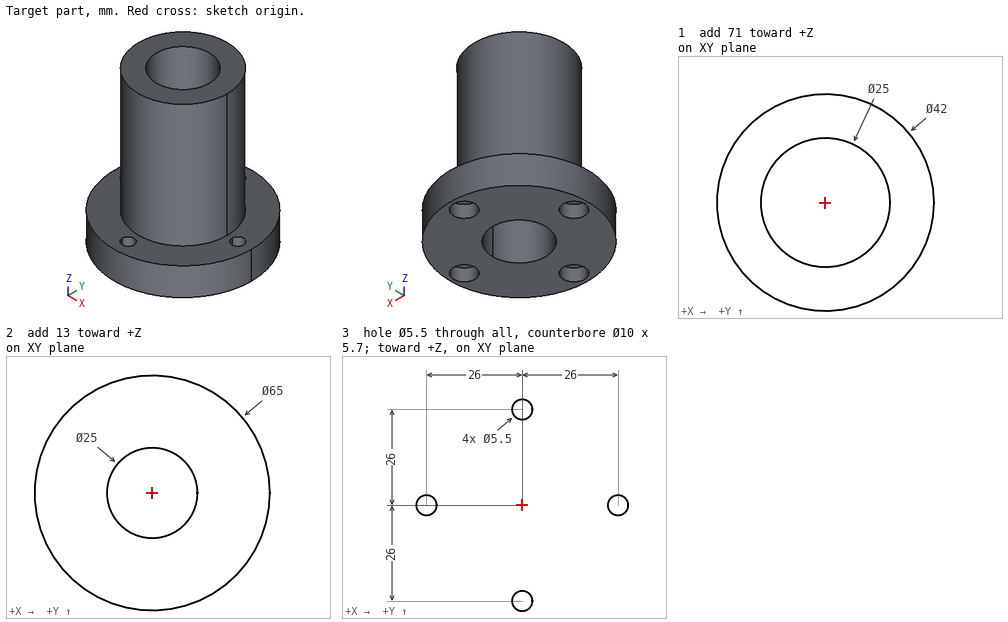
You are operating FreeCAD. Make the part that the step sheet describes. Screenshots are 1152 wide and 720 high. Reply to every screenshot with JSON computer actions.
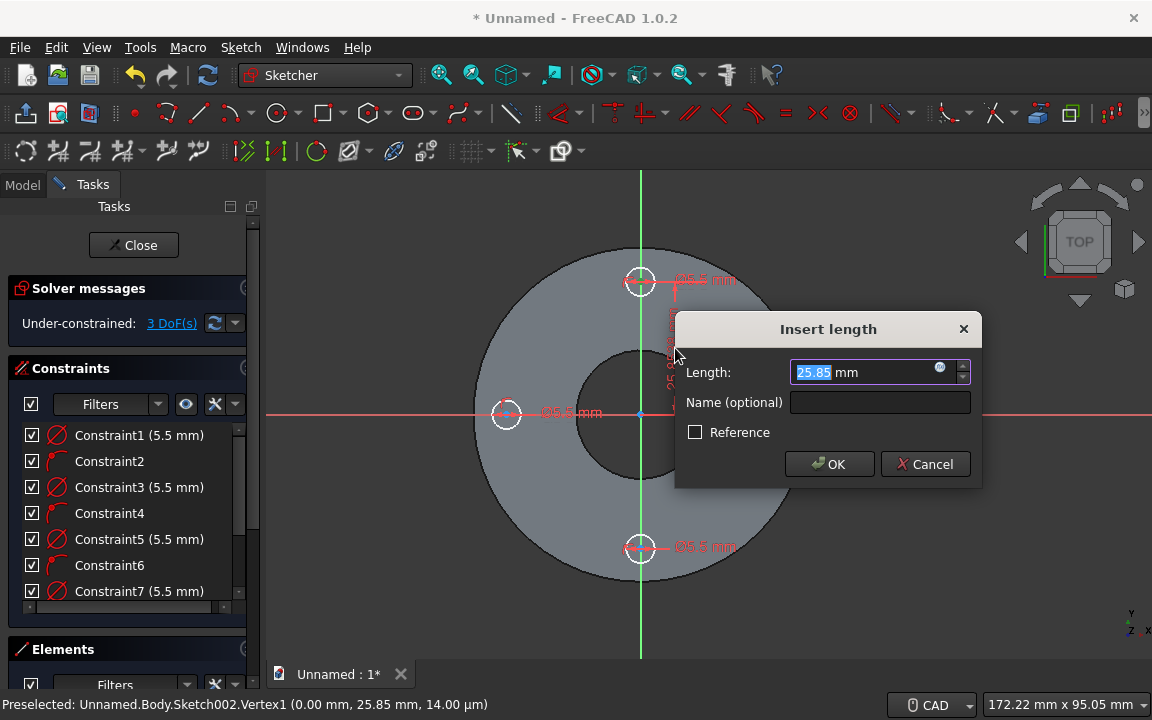
{"action": "type", "text": "26"}
{"action": "key", "text": "Return"}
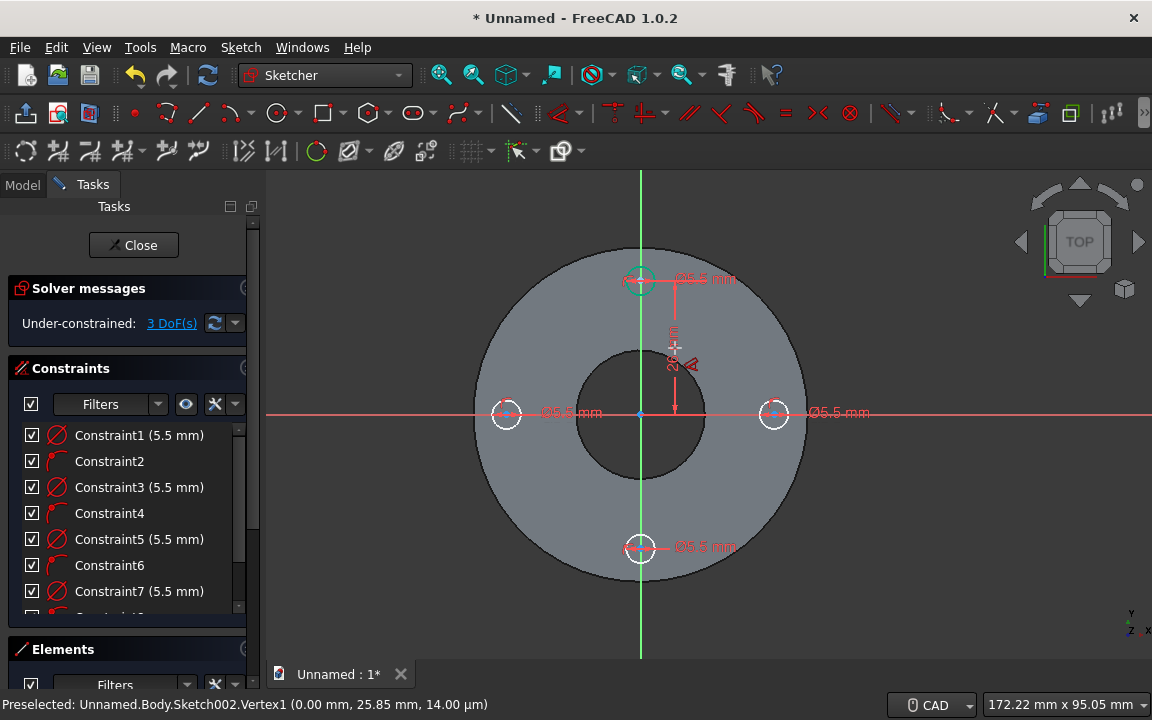
{"action": "left_click", "coordinate": [507, 415]}
{"action": "left_click", "coordinate": [574, 449]}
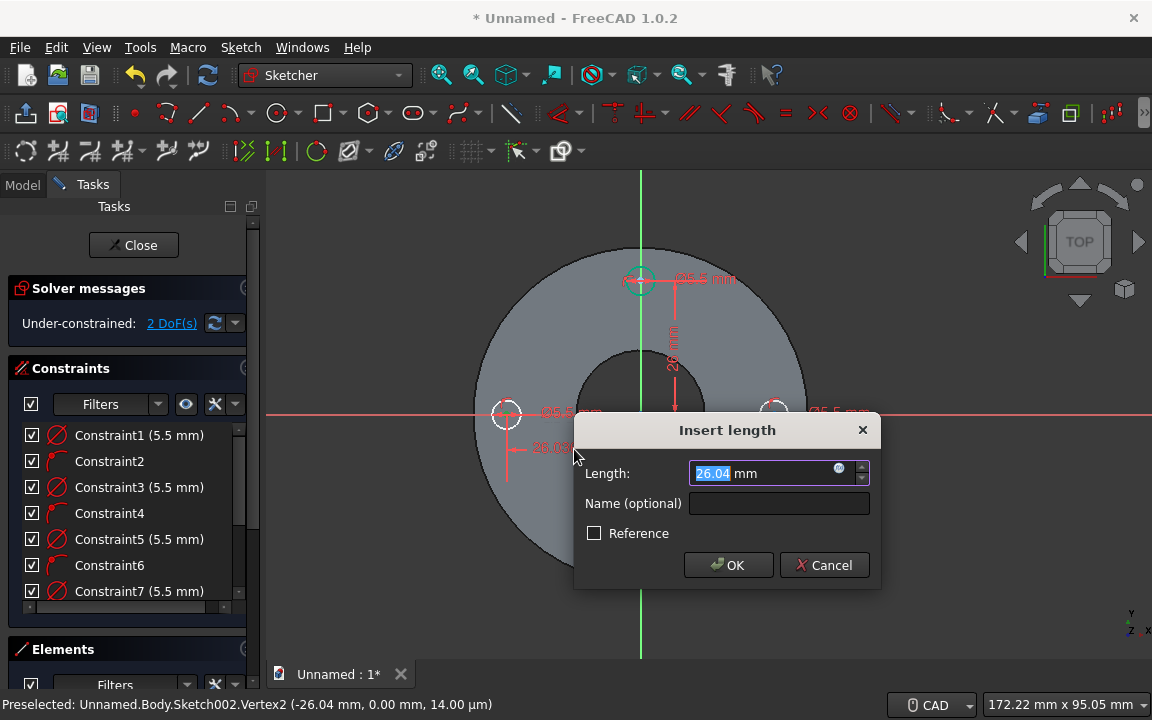
{"action": "type", "text": "26"}
{"action": "key", "text": "Return"}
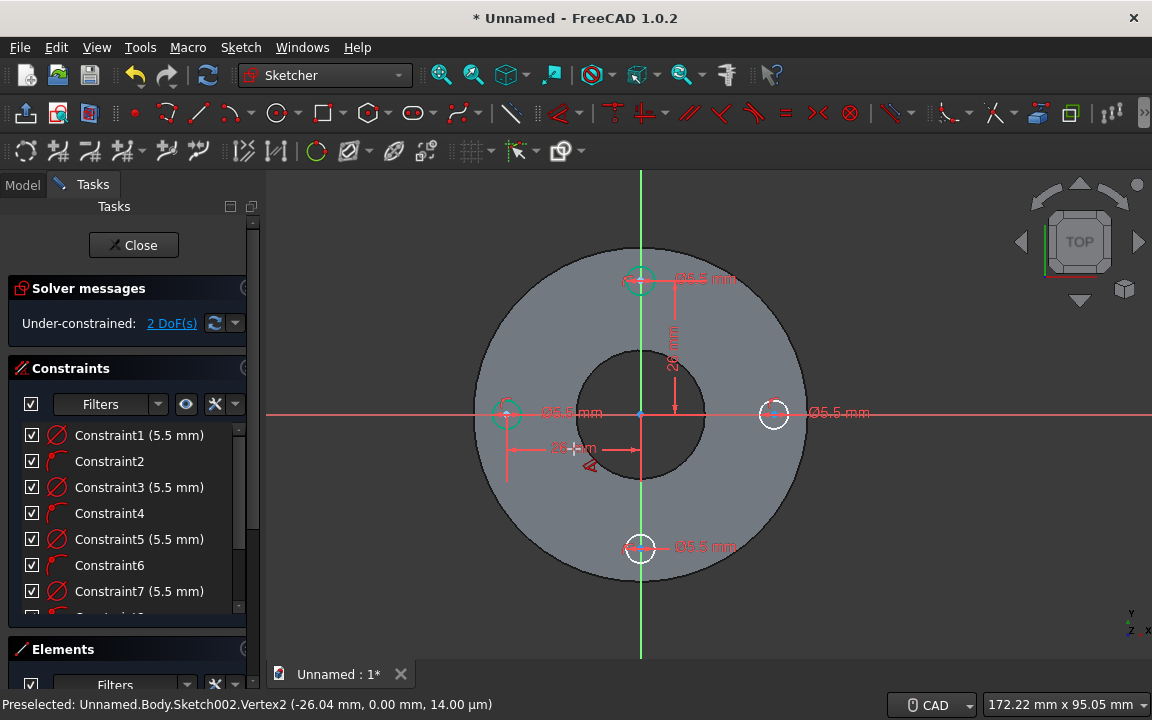
{"action": "left_click", "coordinate": [641, 549]}
{"action": "left_click", "coordinate": [675, 482]}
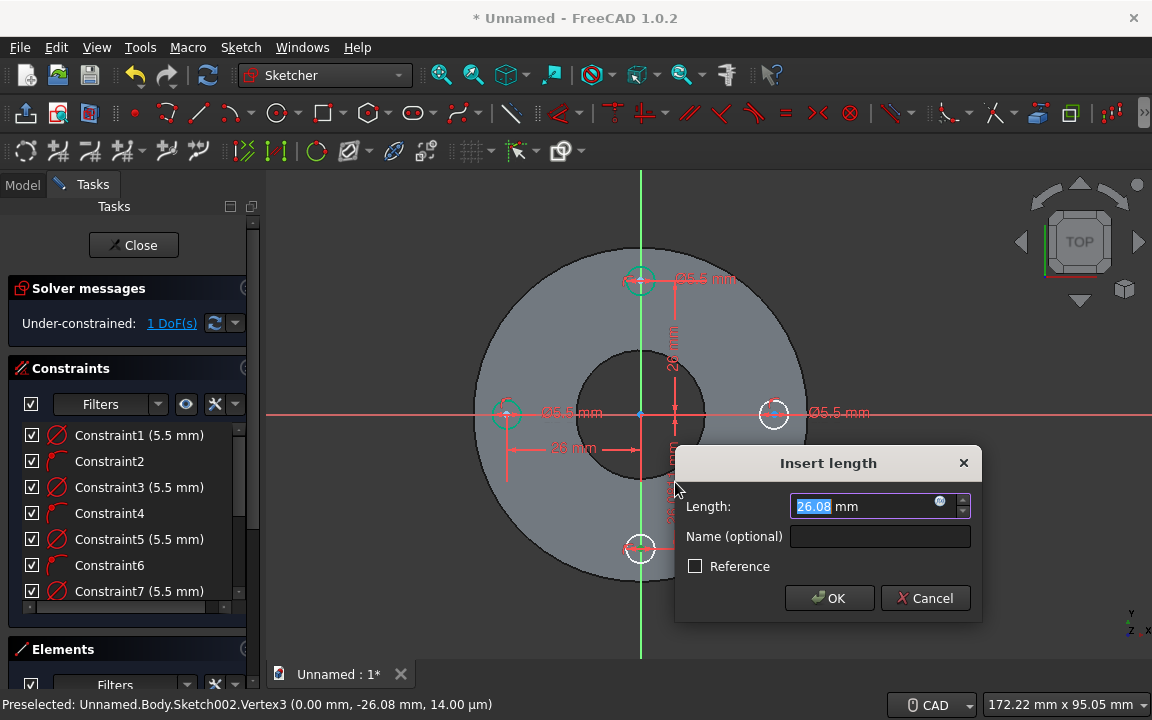
{"action": "type", "text": "26"}
{"action": "key", "text": "Return"}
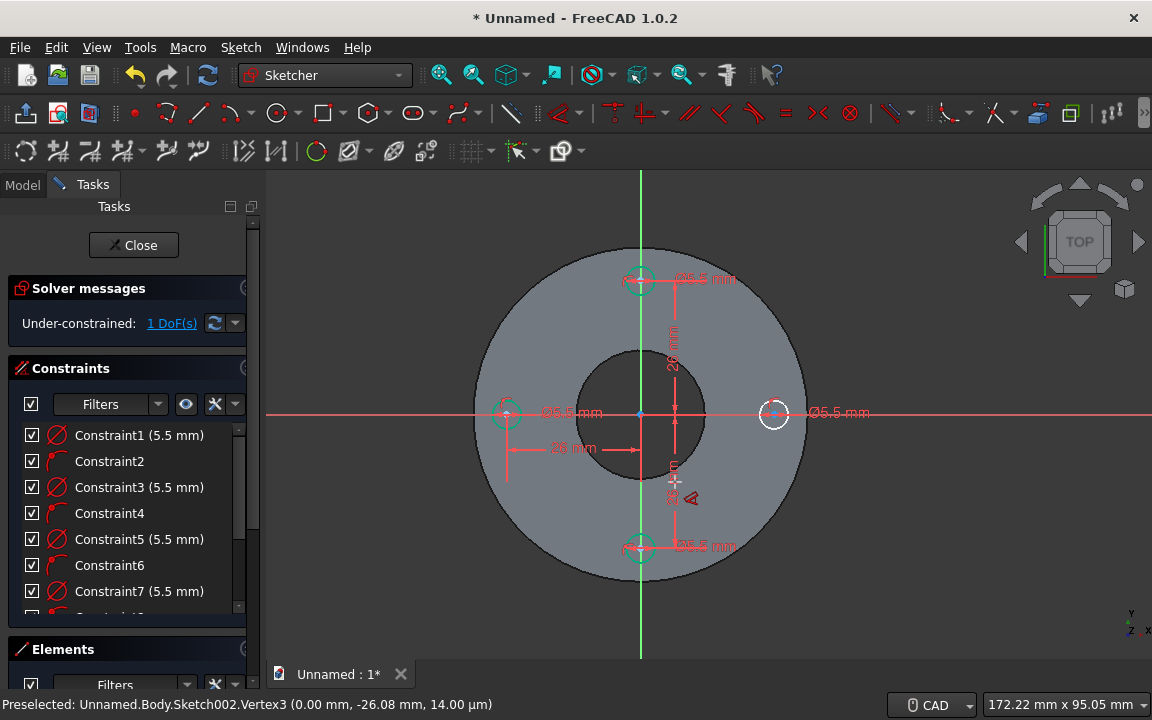
{"action": "left_click", "coordinate": [774, 415]}
{"action": "left_click", "coordinate": [707, 449]}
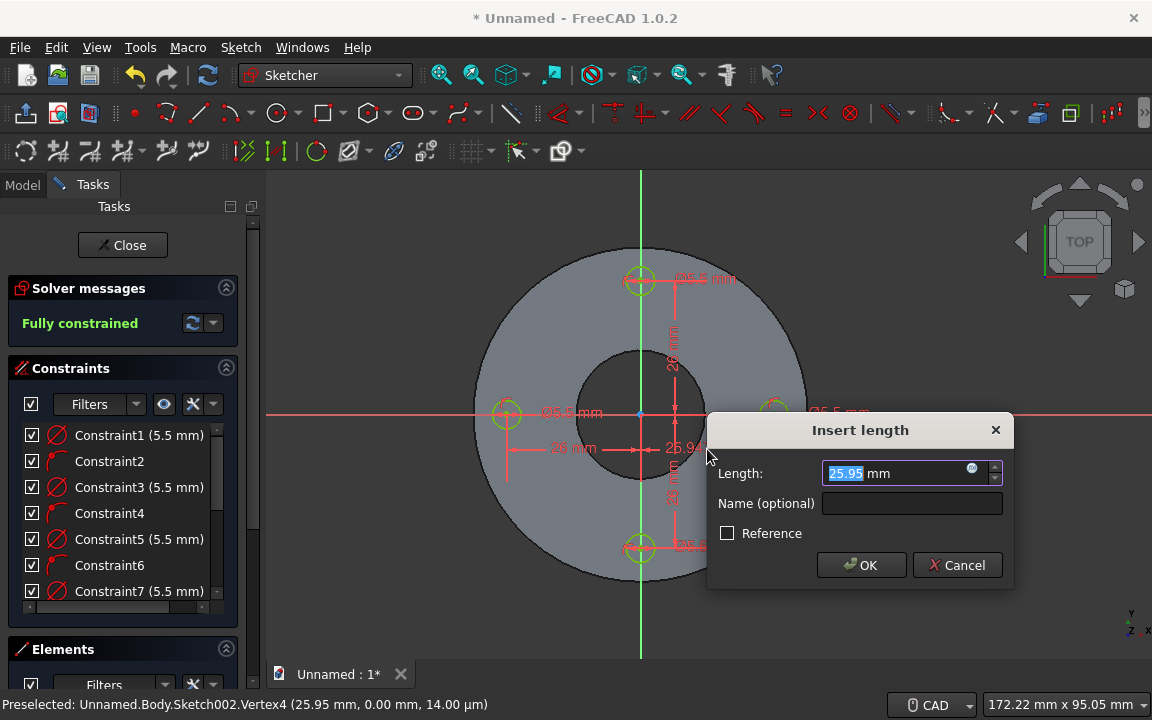
{"action": "type", "text": "26"}
{"action": "key", "text": "Return"}
{"action": "key", "text": "Escape"}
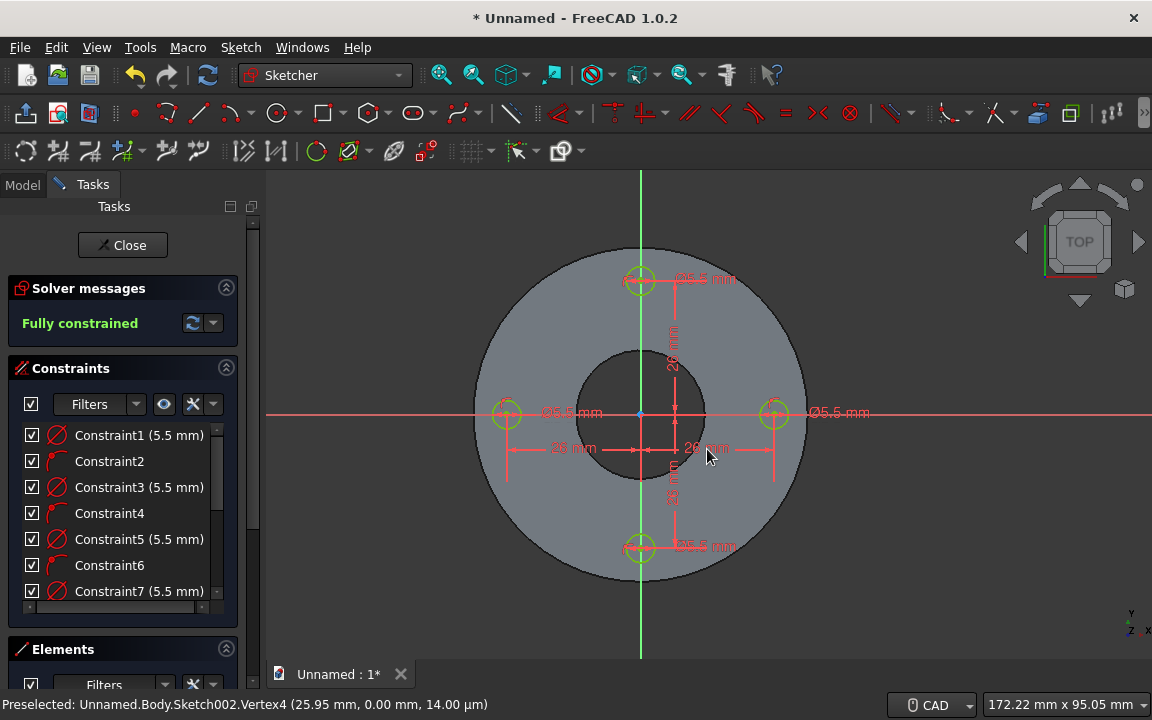
{"action": "left_click", "coordinate": [123, 245]}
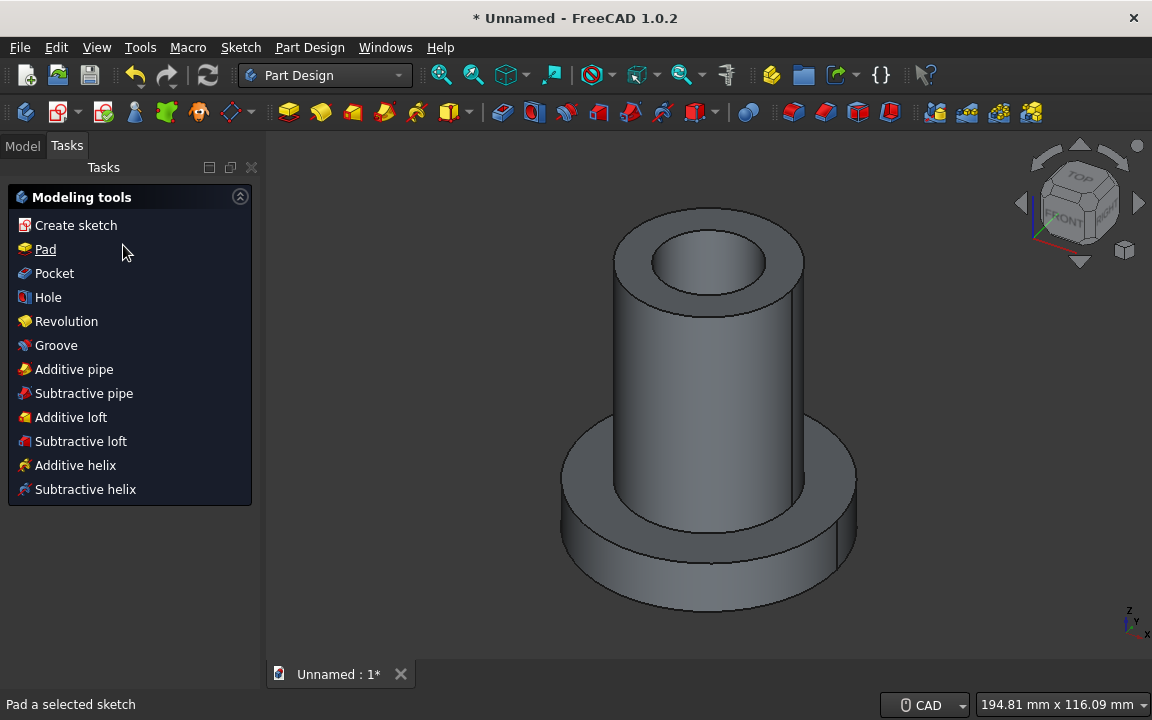
{"action": "left_click", "coordinate": [536, 112]}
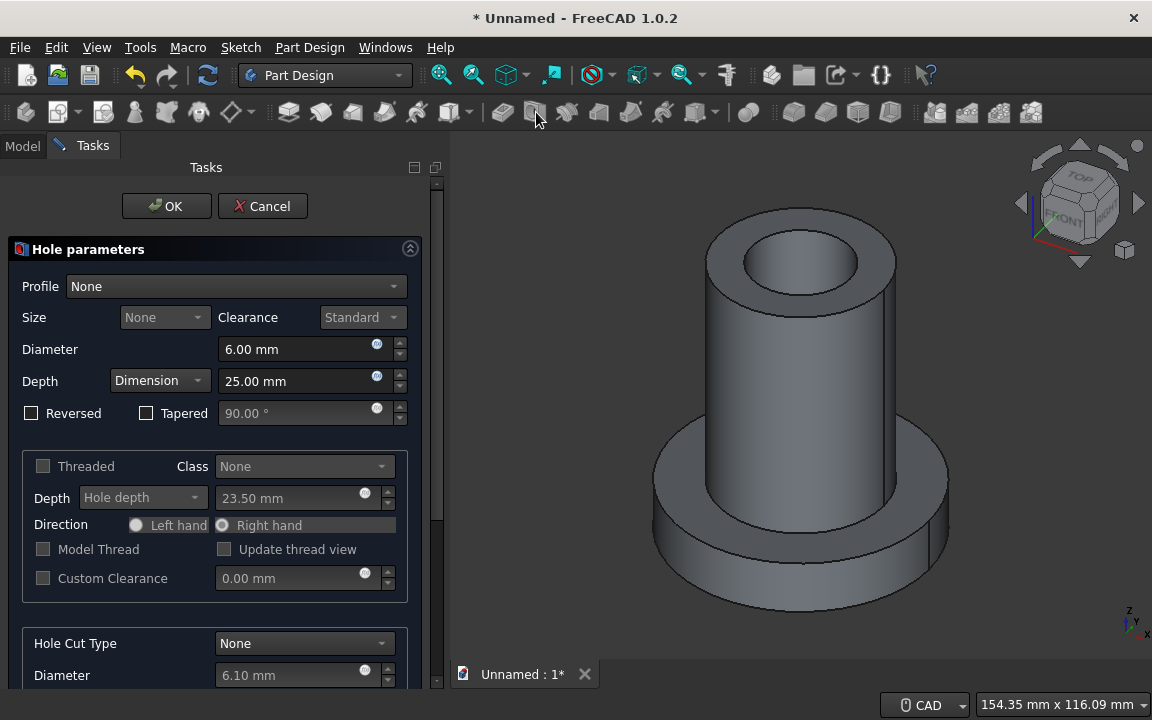
{"action": "triple_click", "coordinate": [305, 349]}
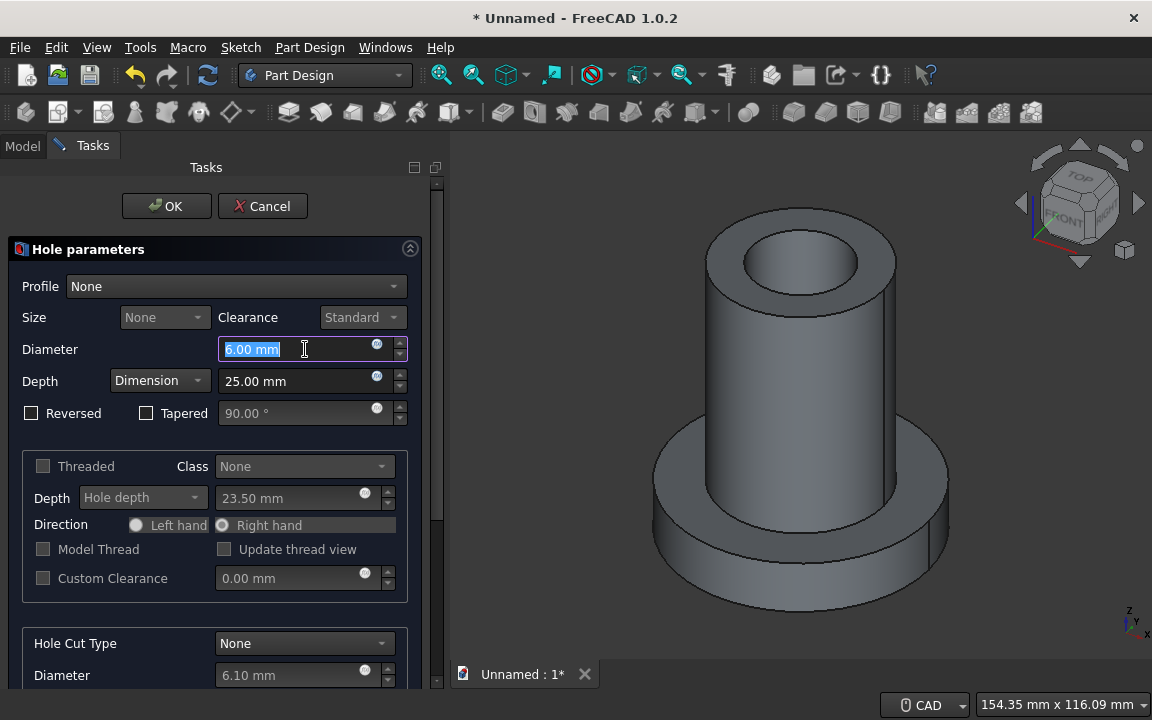
{"action": "type", "text": "5.5"}
{"action": "key", "text": "Tab"}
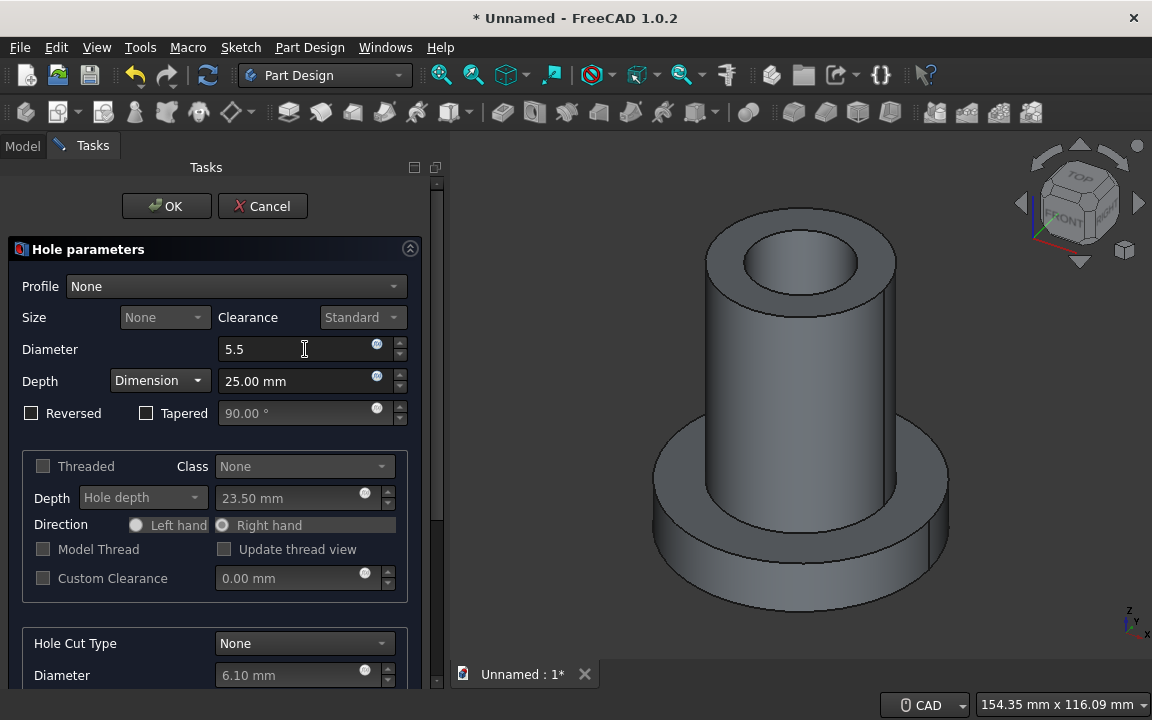
{"action": "left_click", "coordinate": [161, 380]}